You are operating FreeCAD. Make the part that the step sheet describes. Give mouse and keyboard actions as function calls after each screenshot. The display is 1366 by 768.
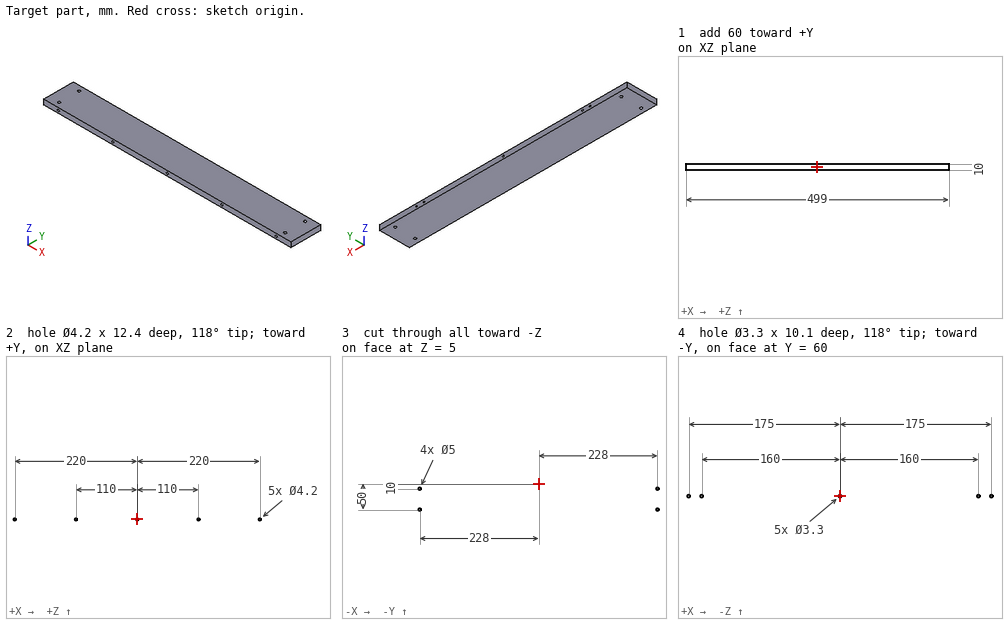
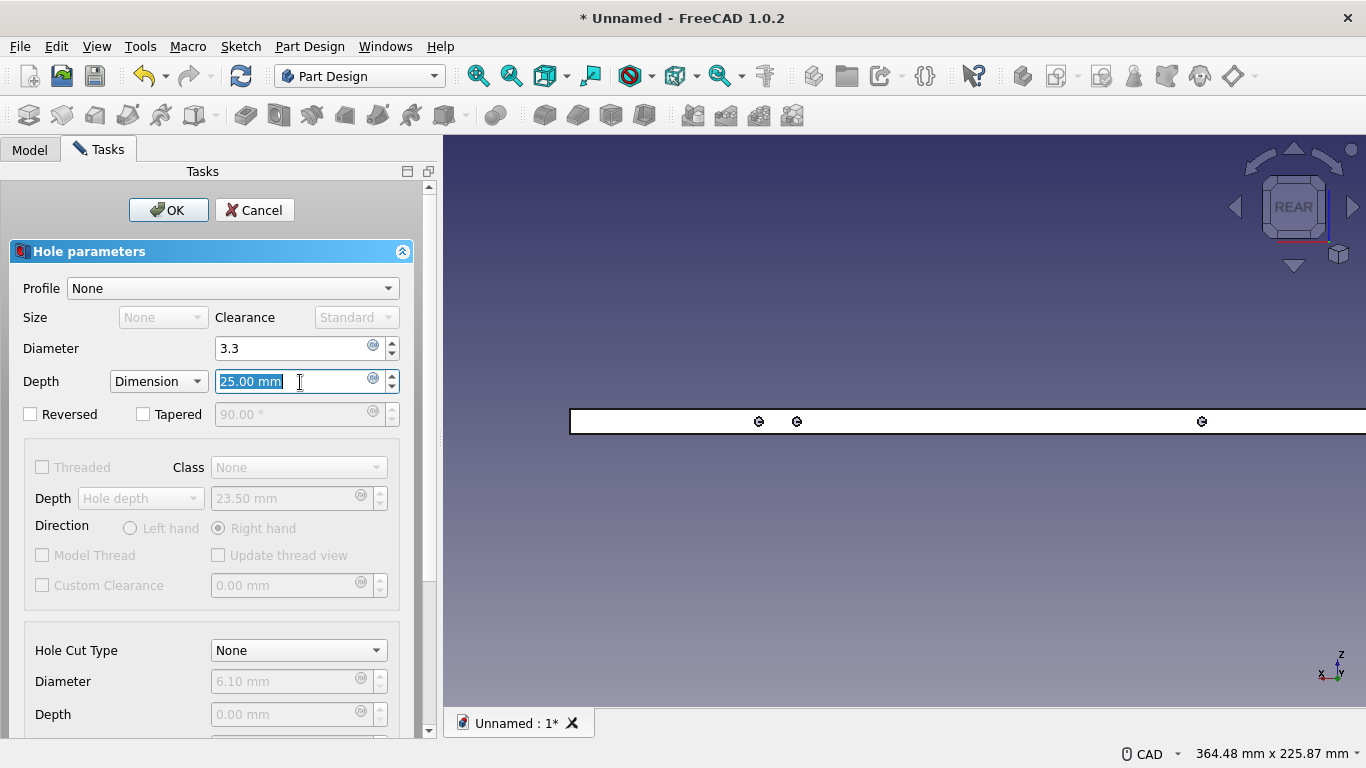
text(10.1)
key(Tab)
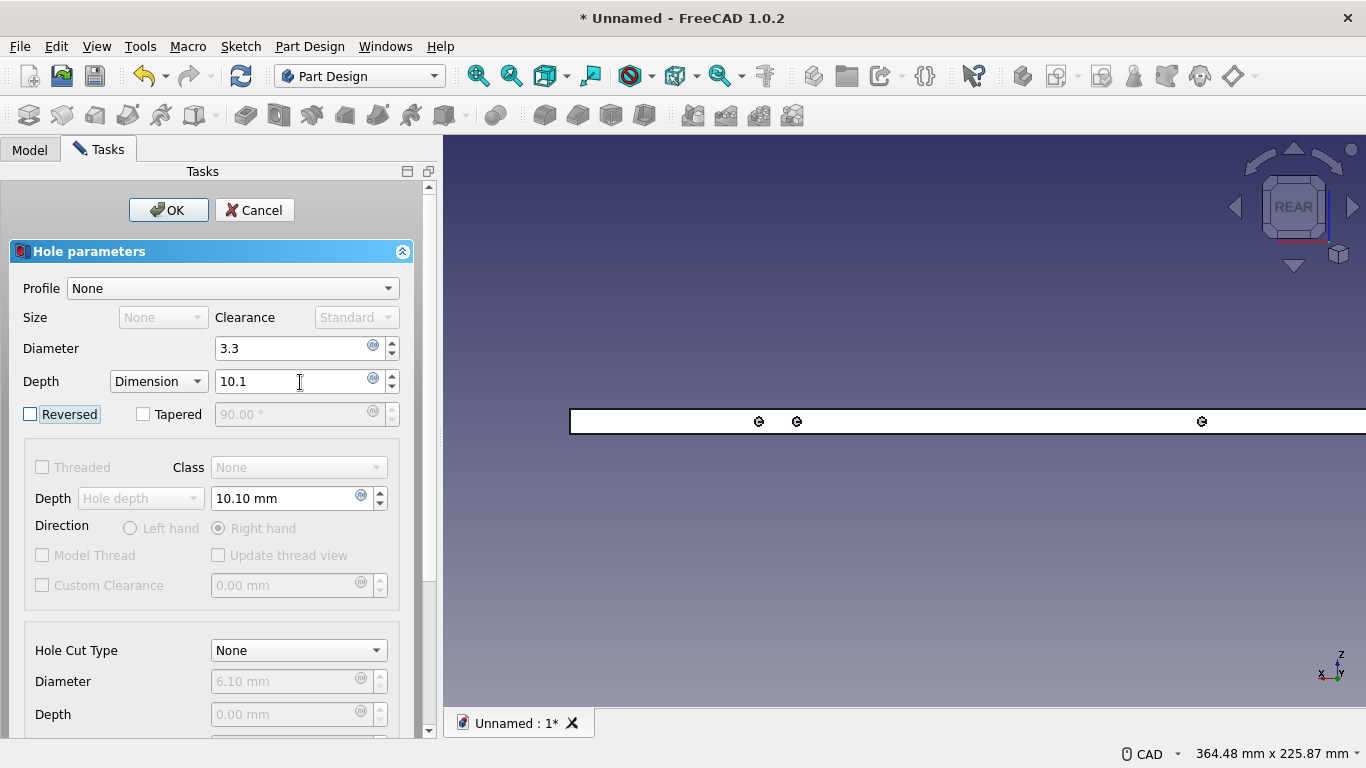
click(169, 210)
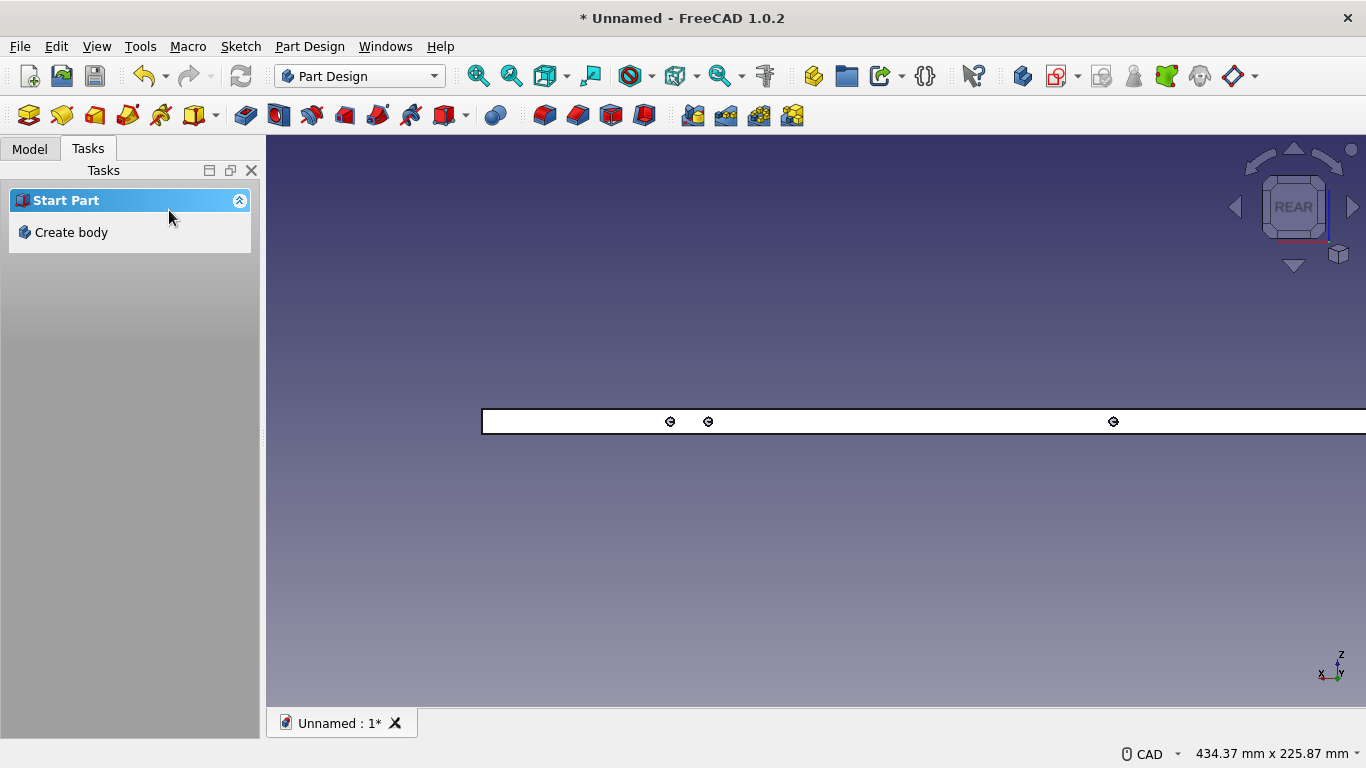
key(0)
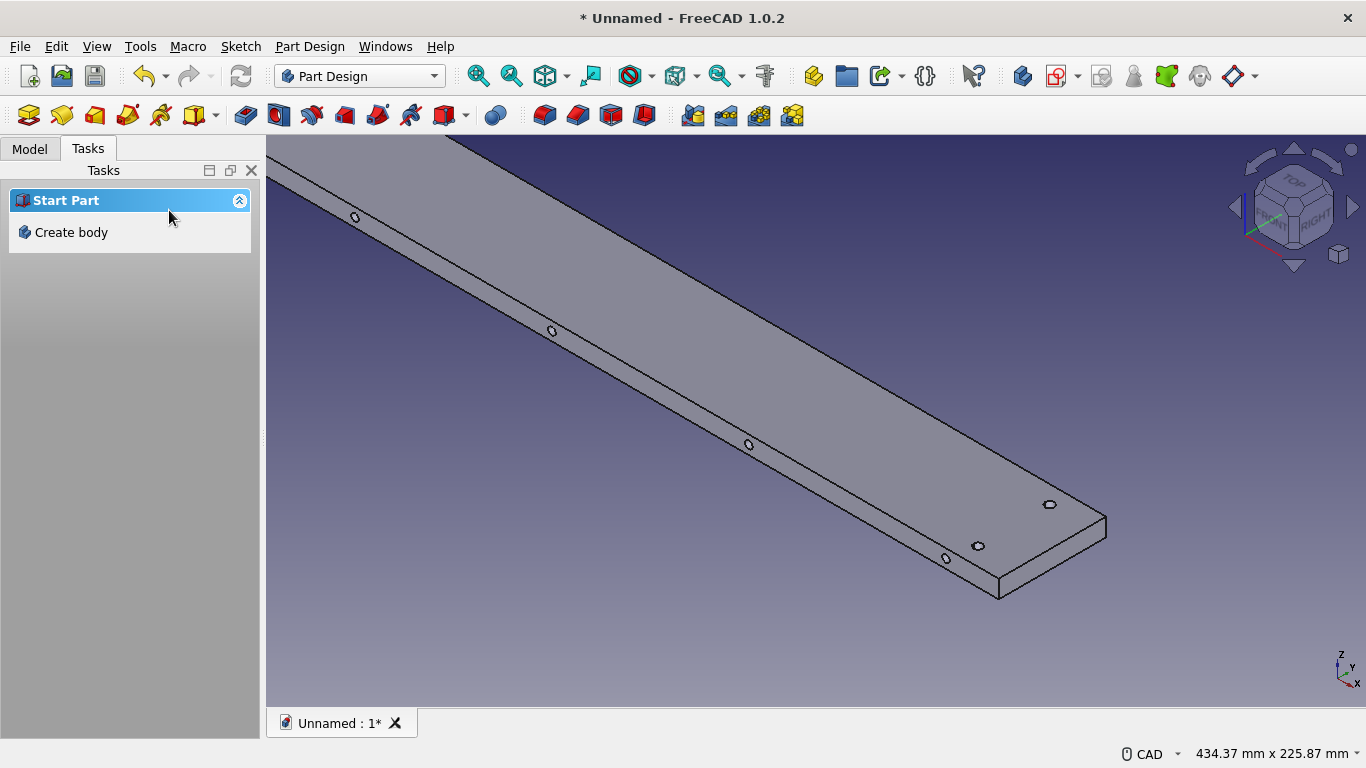
key(v)
key(f)